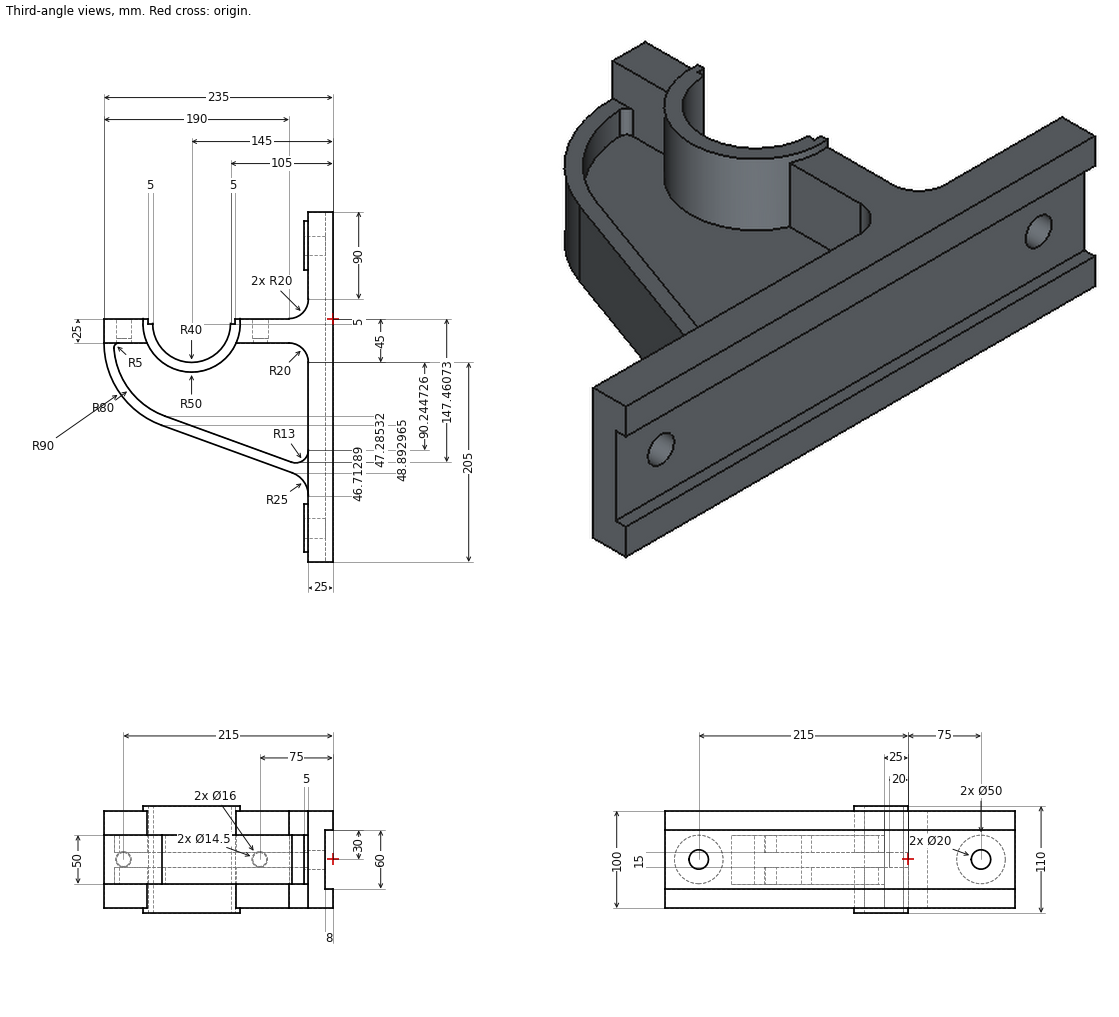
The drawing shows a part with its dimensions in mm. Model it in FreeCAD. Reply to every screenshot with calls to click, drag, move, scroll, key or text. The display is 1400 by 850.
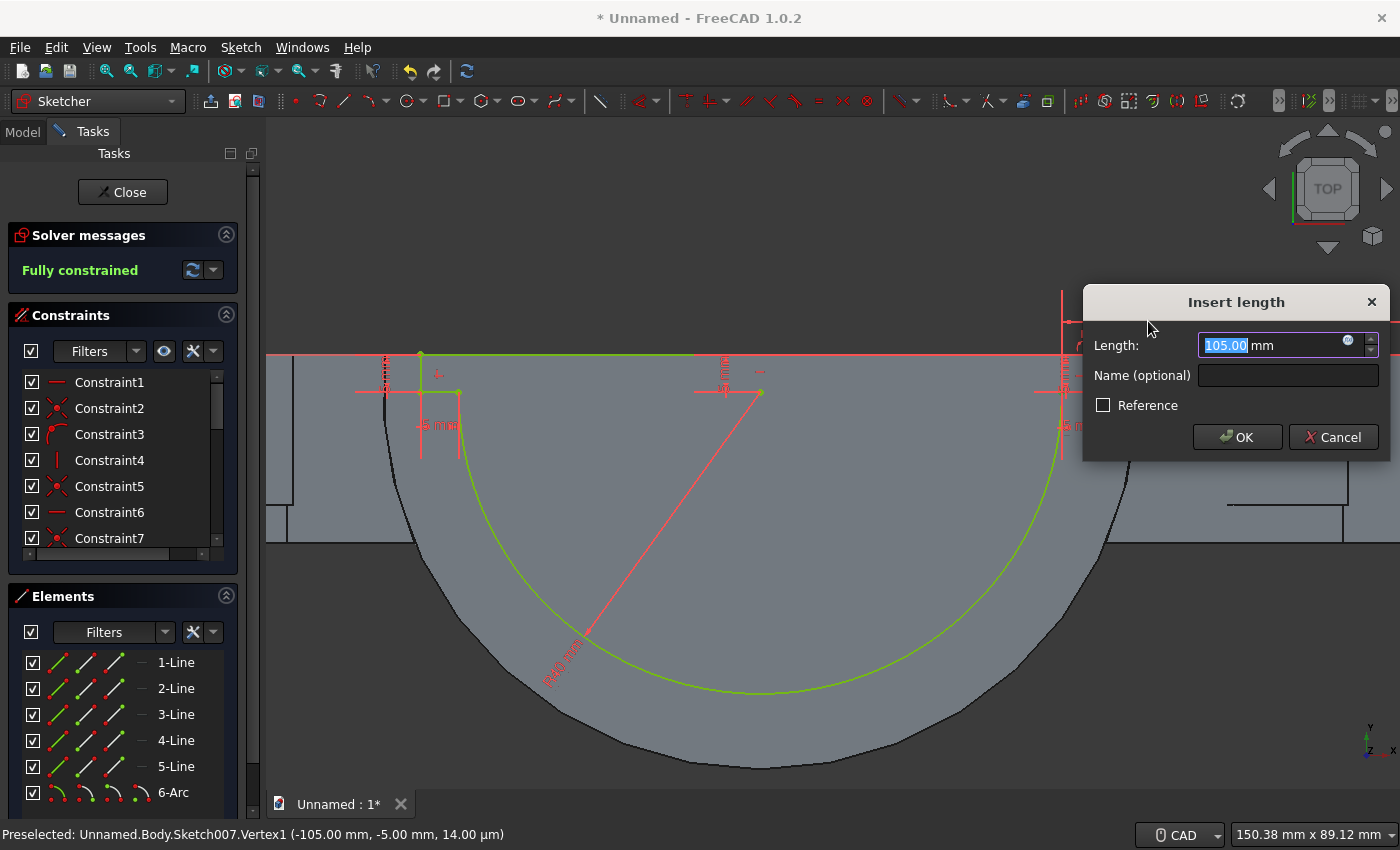
text(105)
key(Return)
key(Escape)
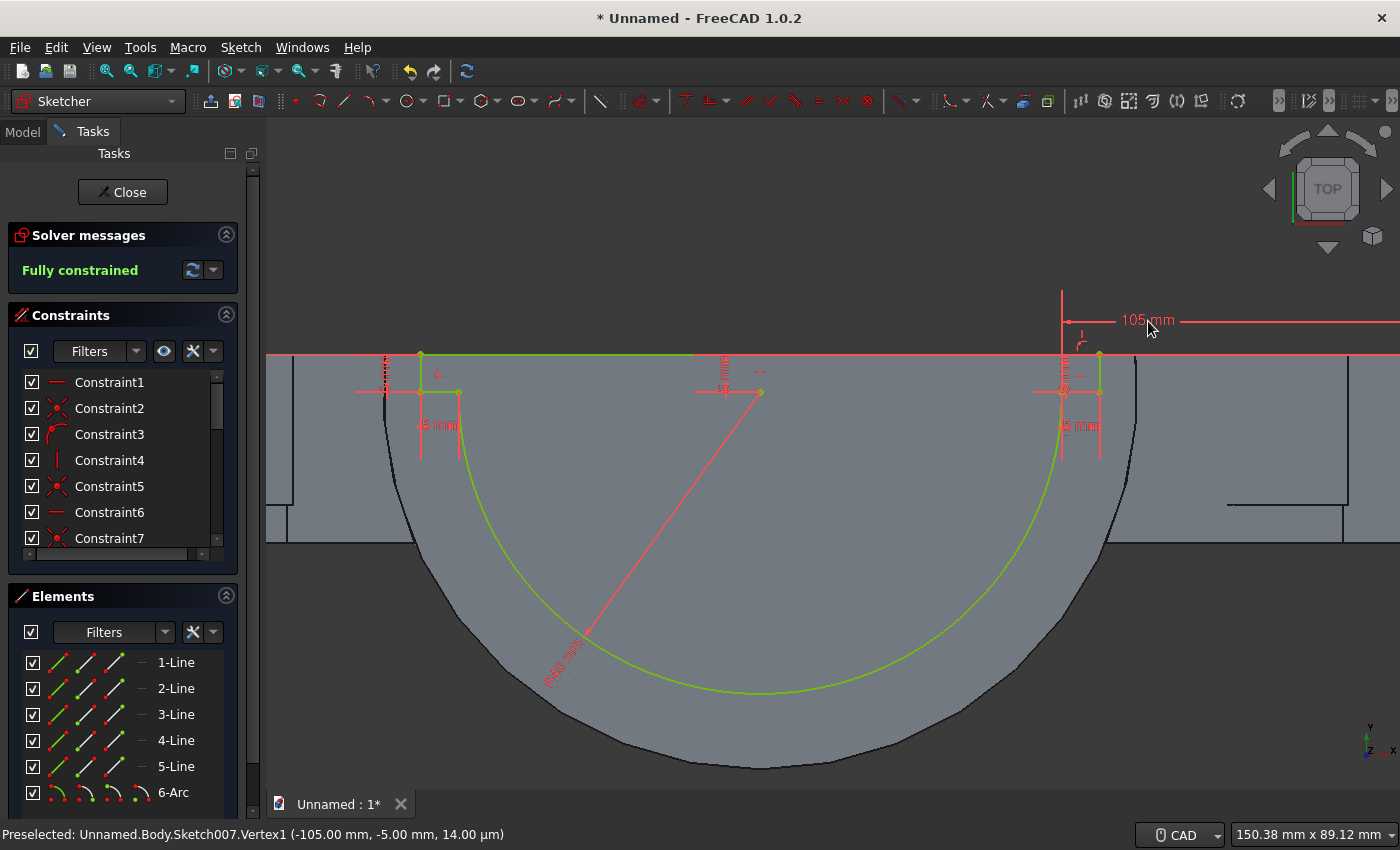
click(123, 192)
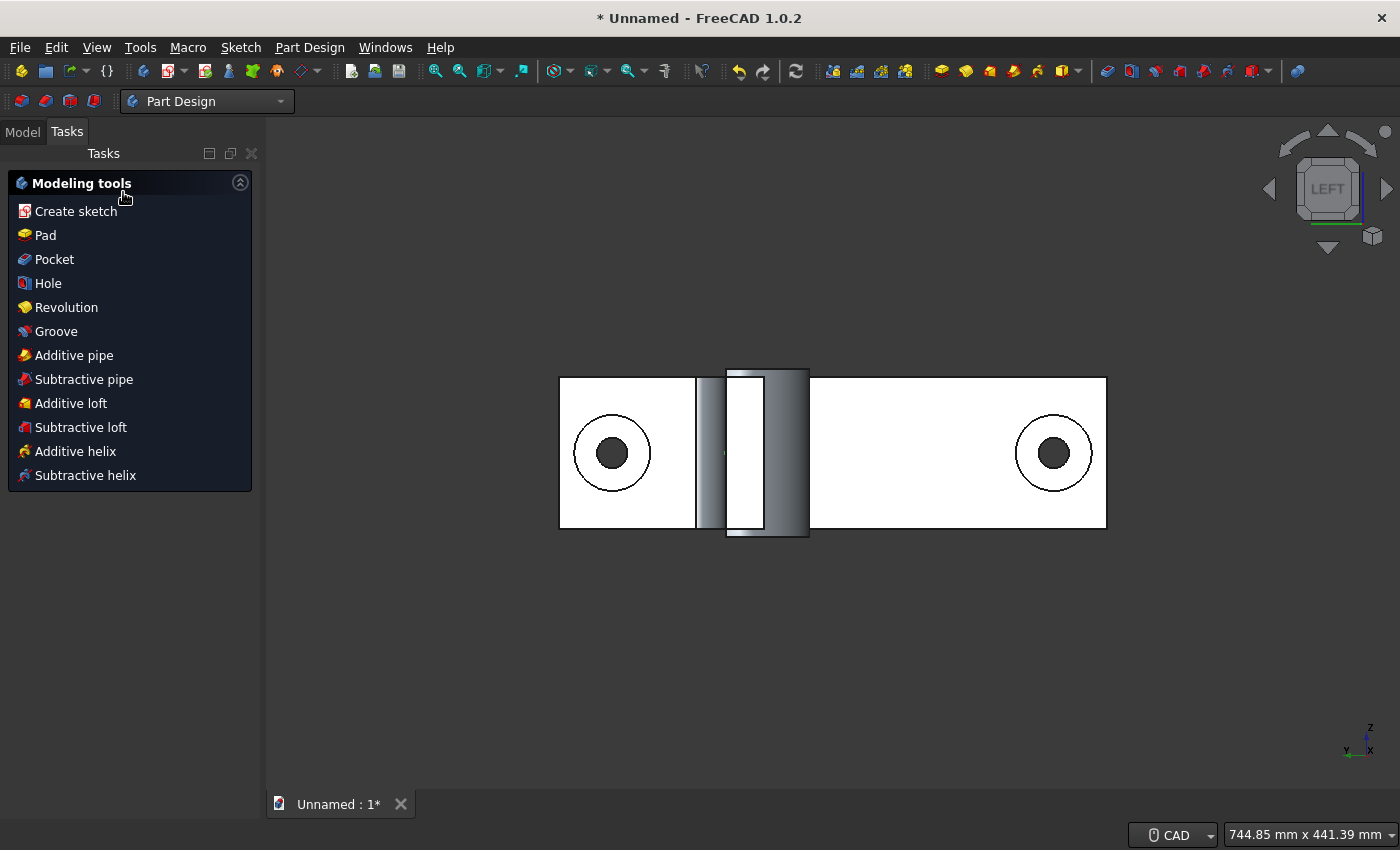
click(1108, 72)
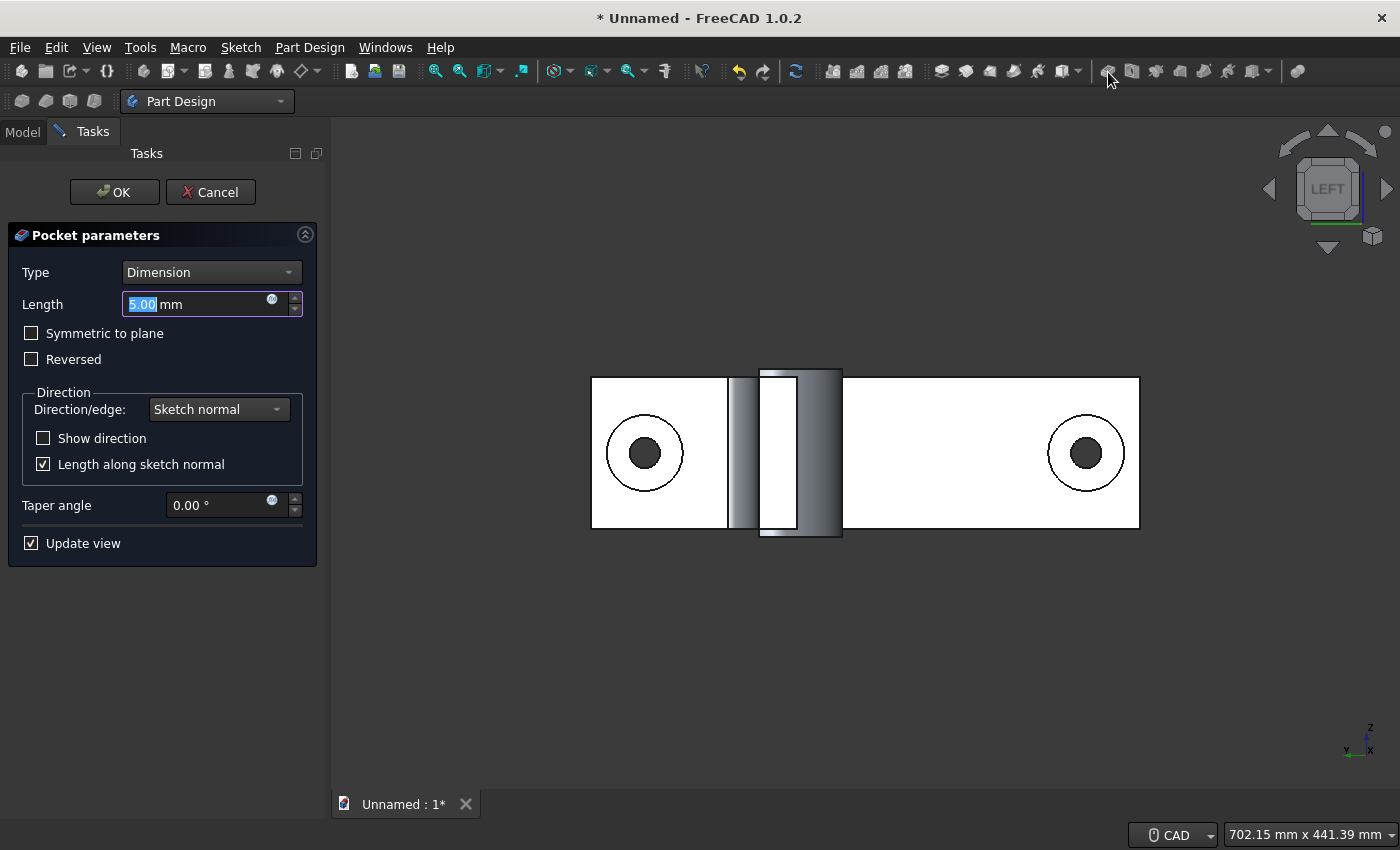
text(110)
key(Tab)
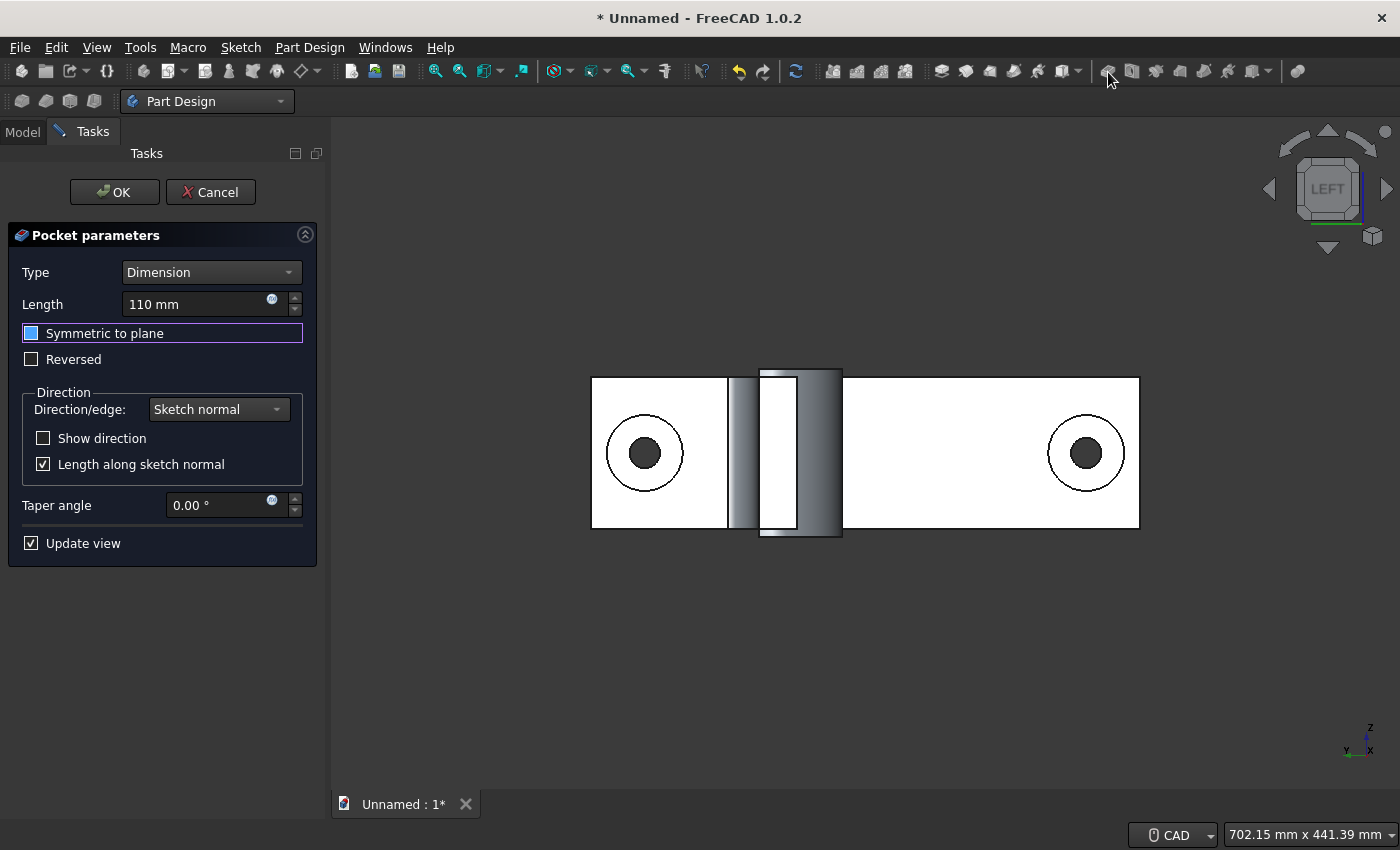
click(30, 333)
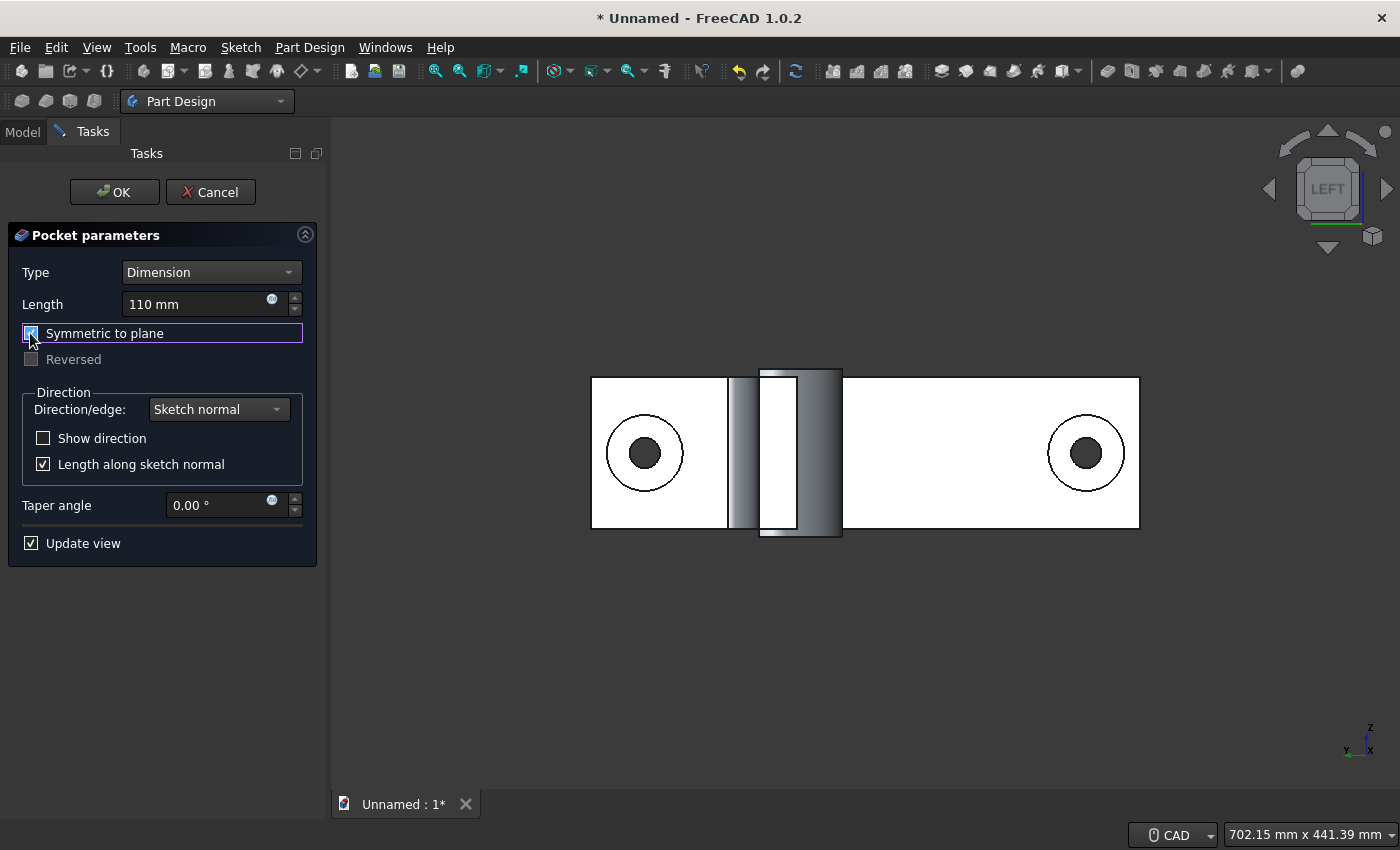
click(115, 192)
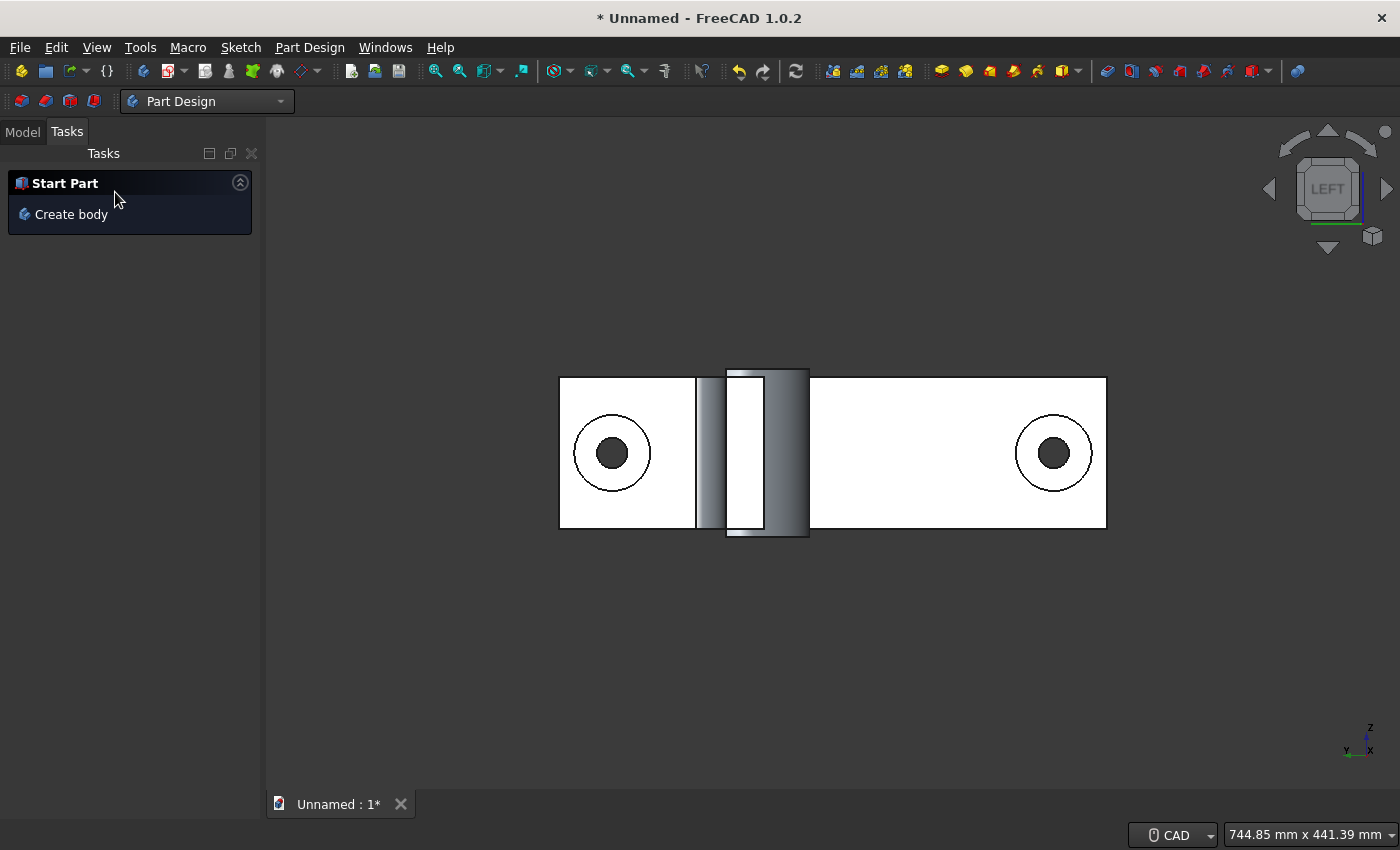
click(168, 72)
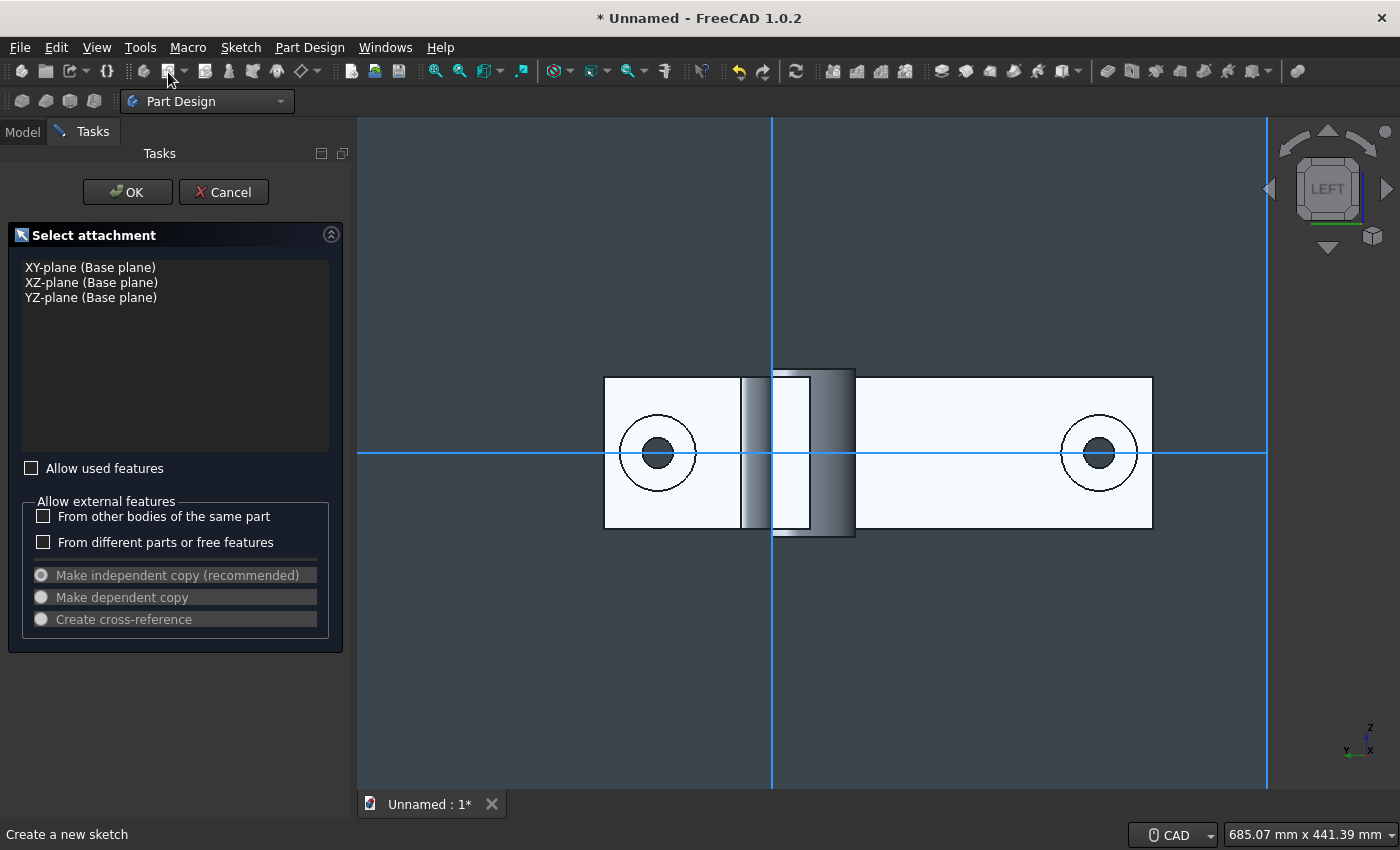
click(82, 268)